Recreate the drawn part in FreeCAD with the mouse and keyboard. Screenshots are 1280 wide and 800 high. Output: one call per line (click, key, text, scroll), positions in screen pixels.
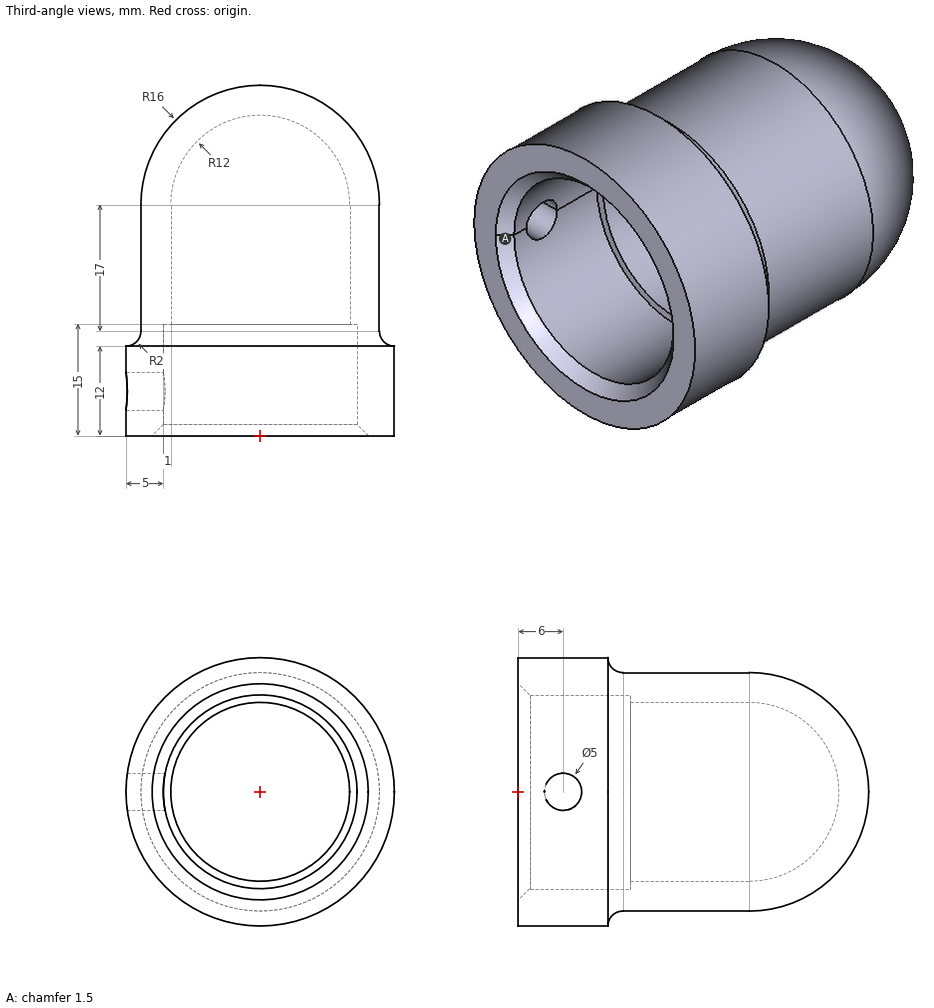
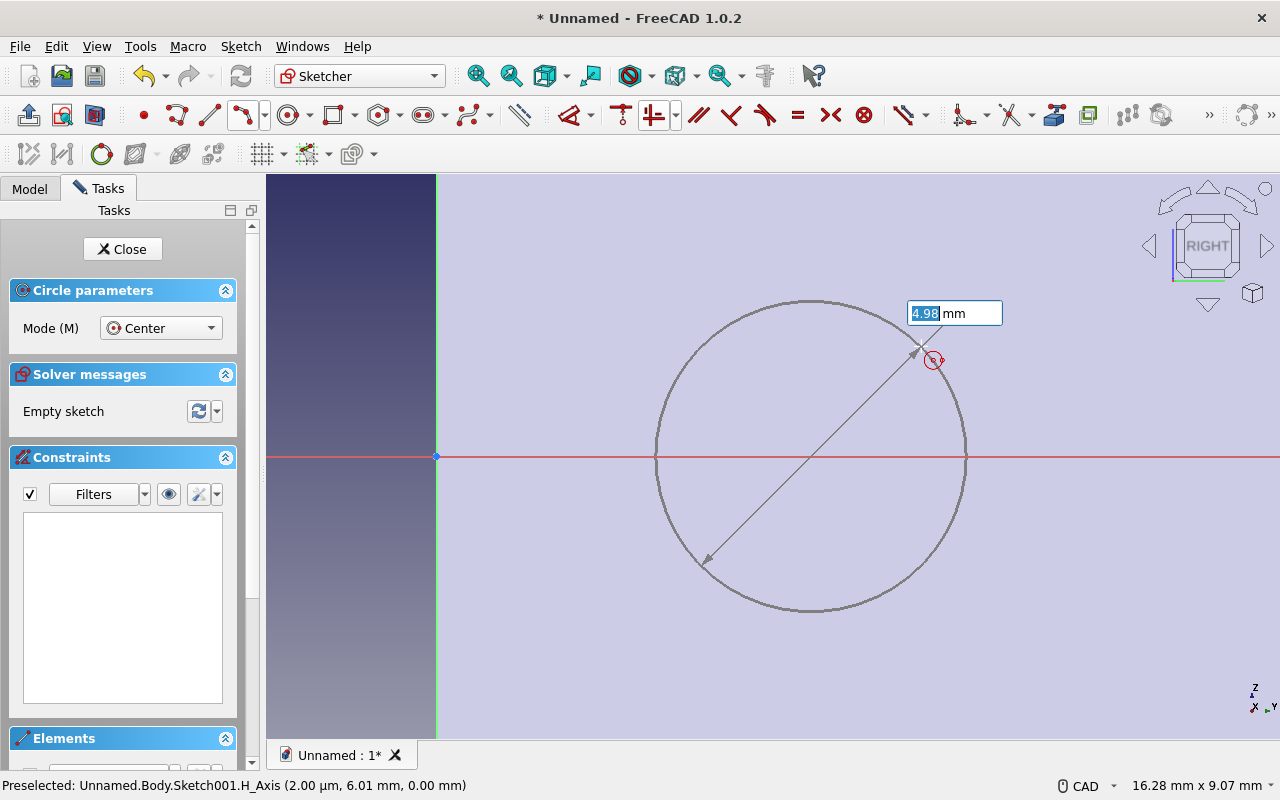
text(5)
key(Return)
key(Escape)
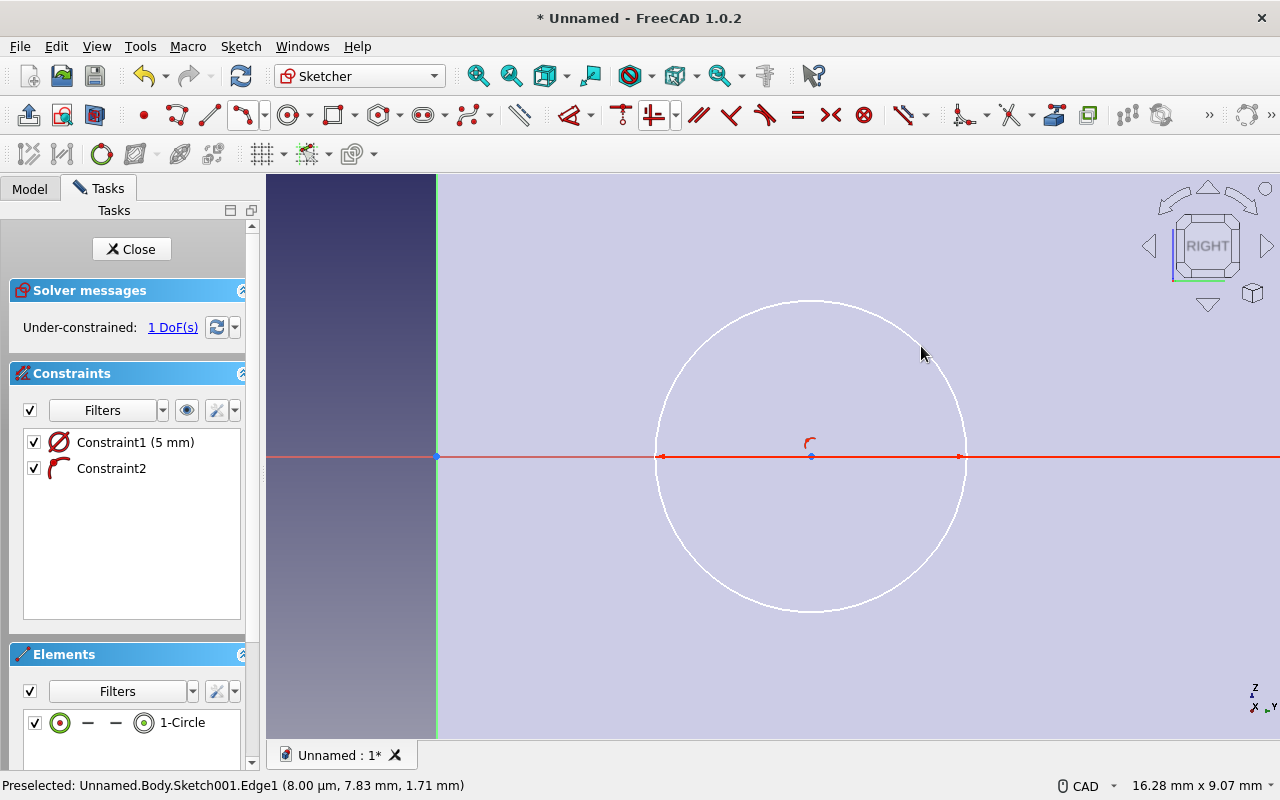
click(568, 116)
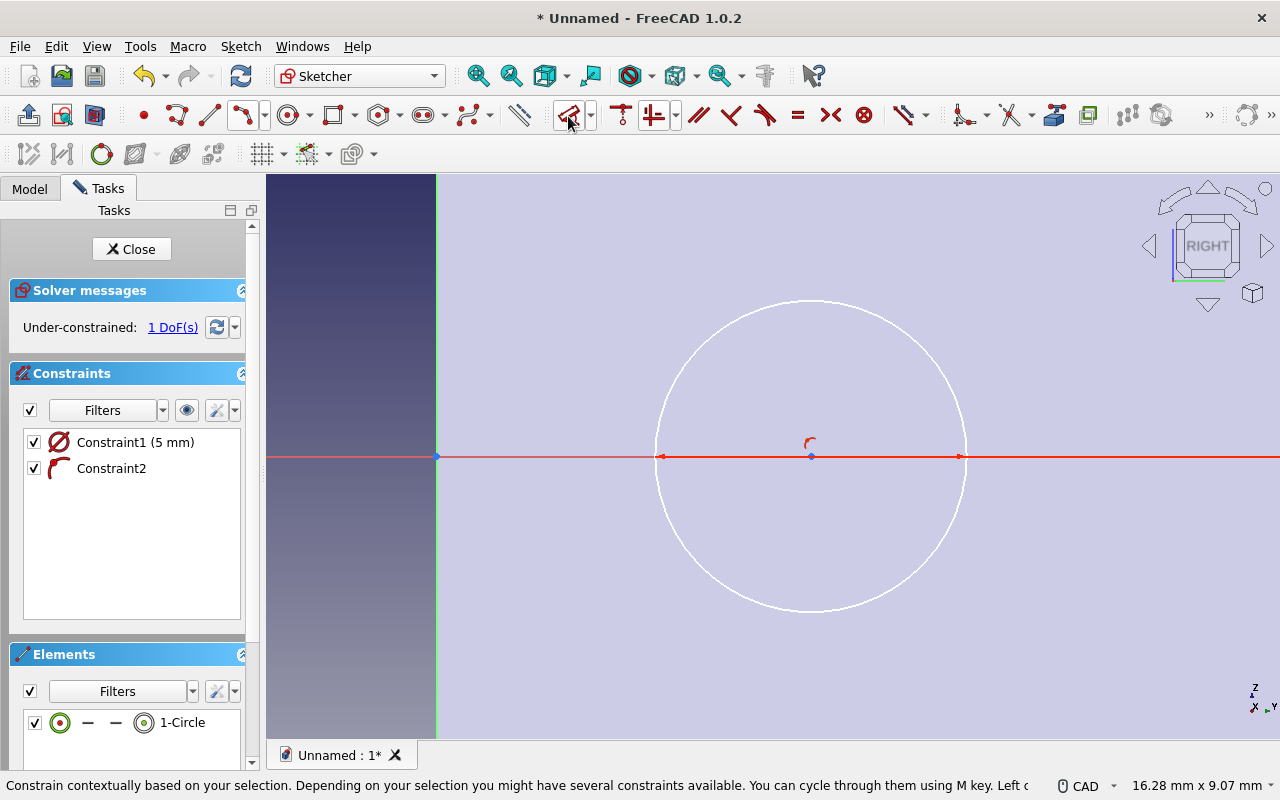
click(811, 456)
click(624, 490)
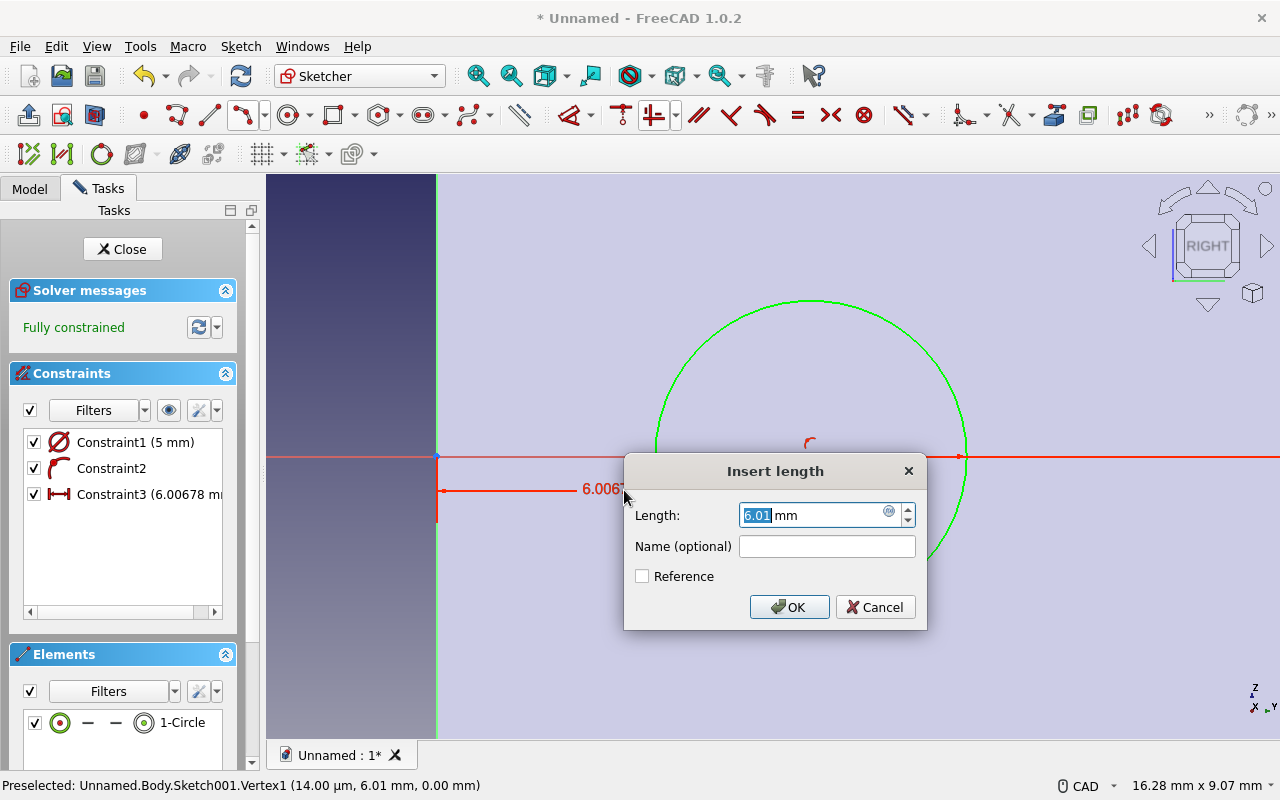
text(6)
key(Return)
key(Escape)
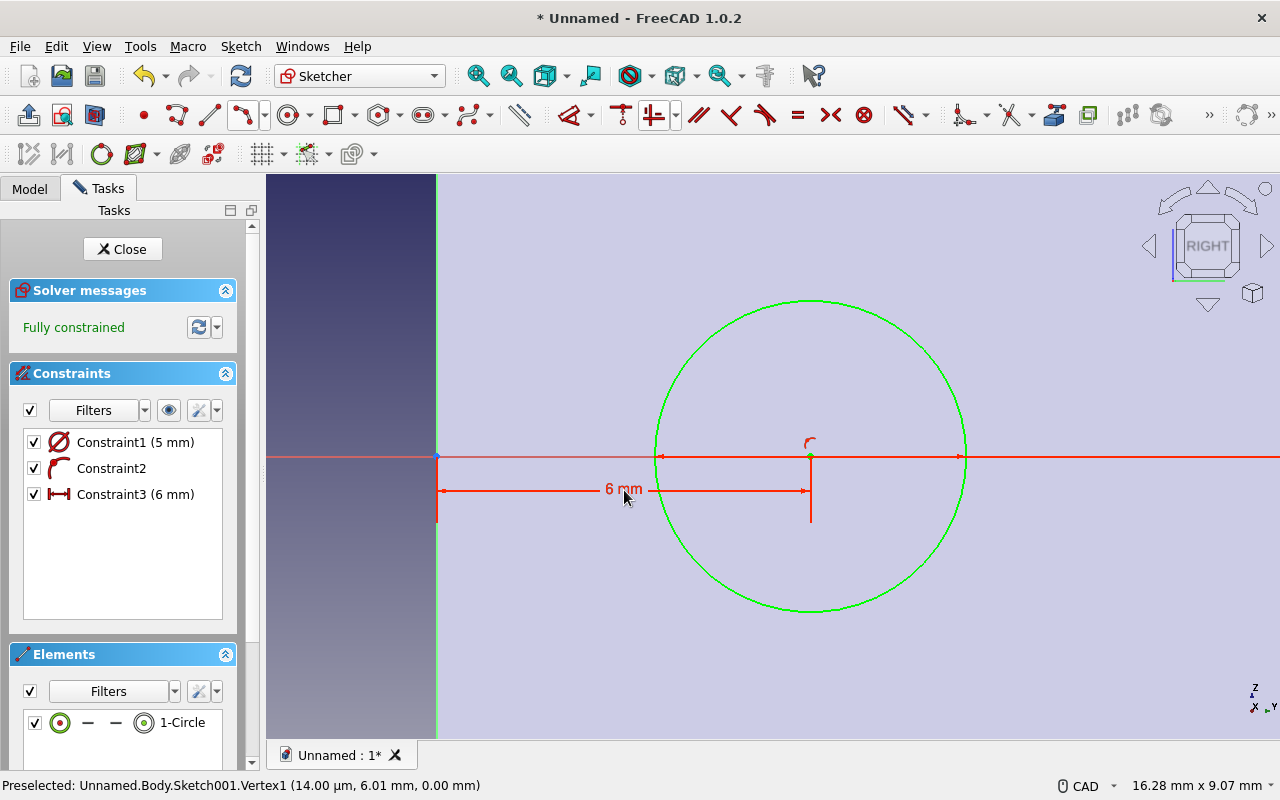
click(123, 249)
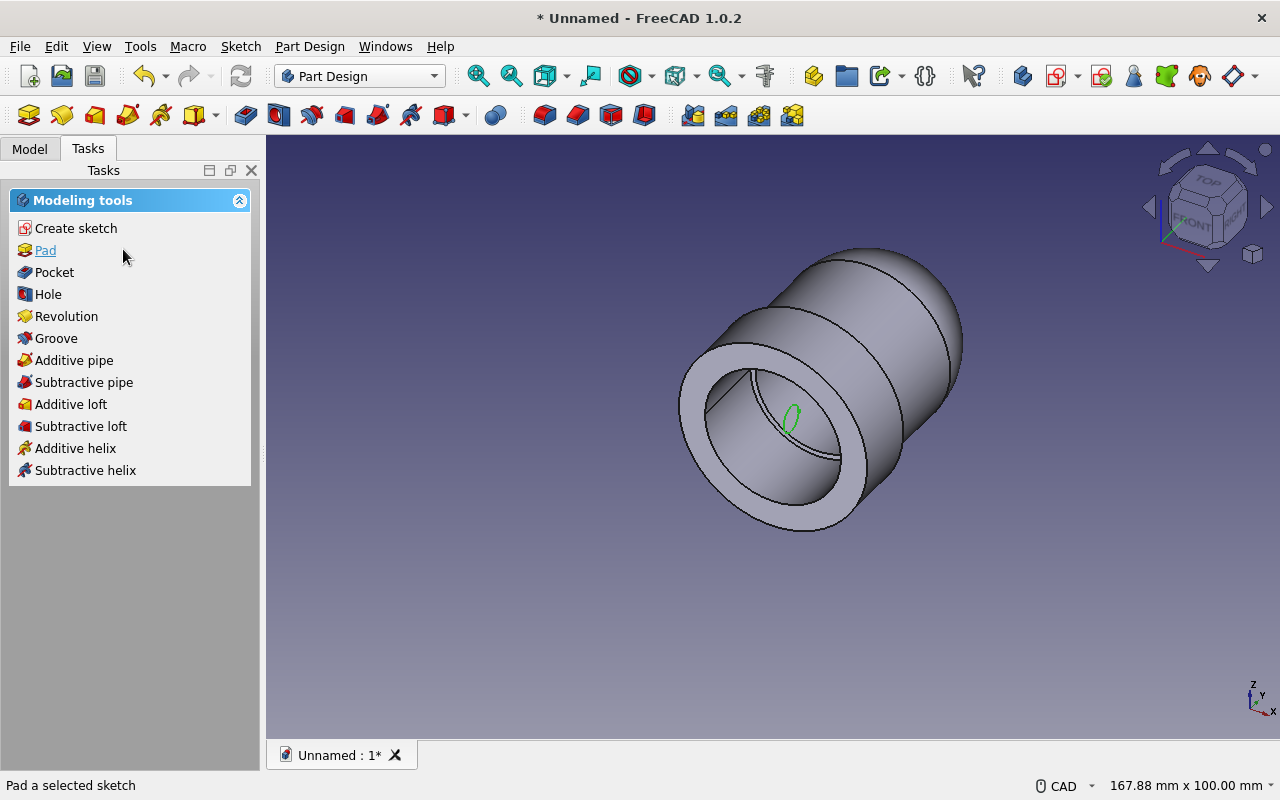
click(246, 116)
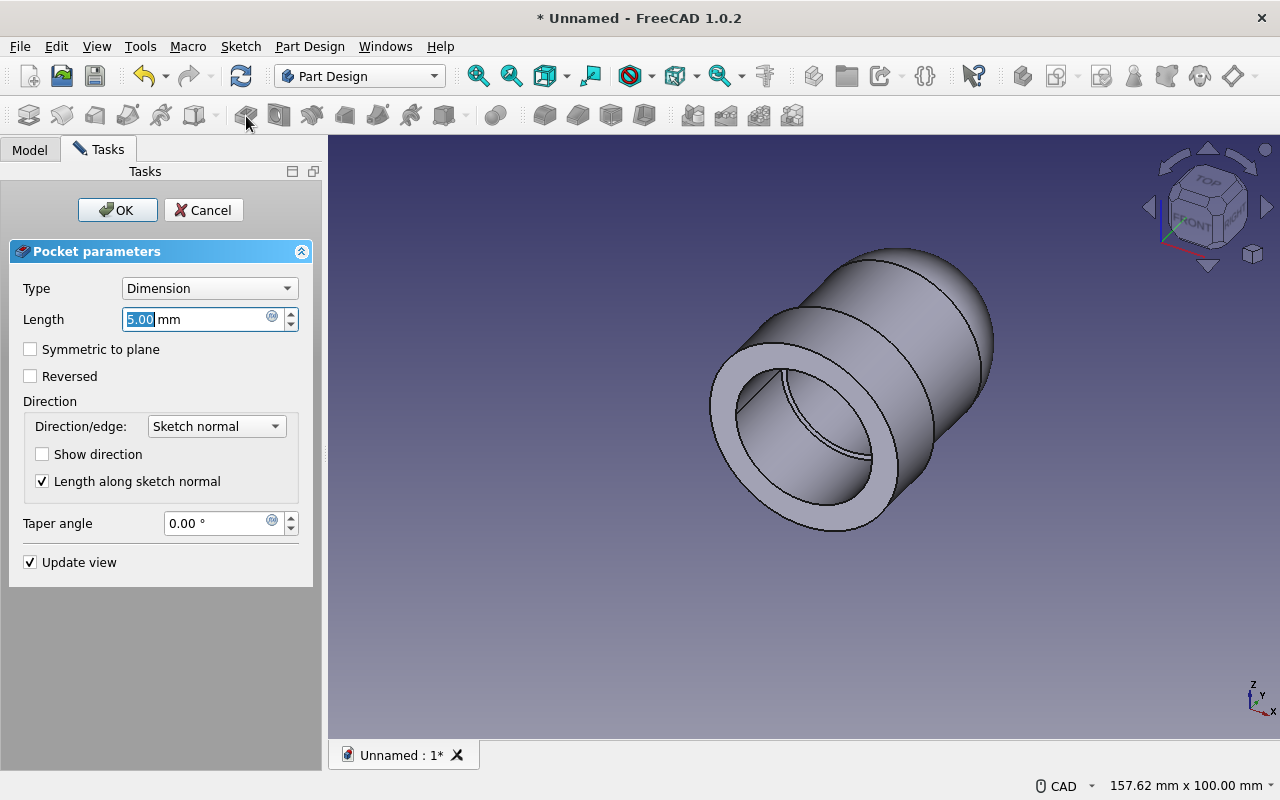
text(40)
key(Tab)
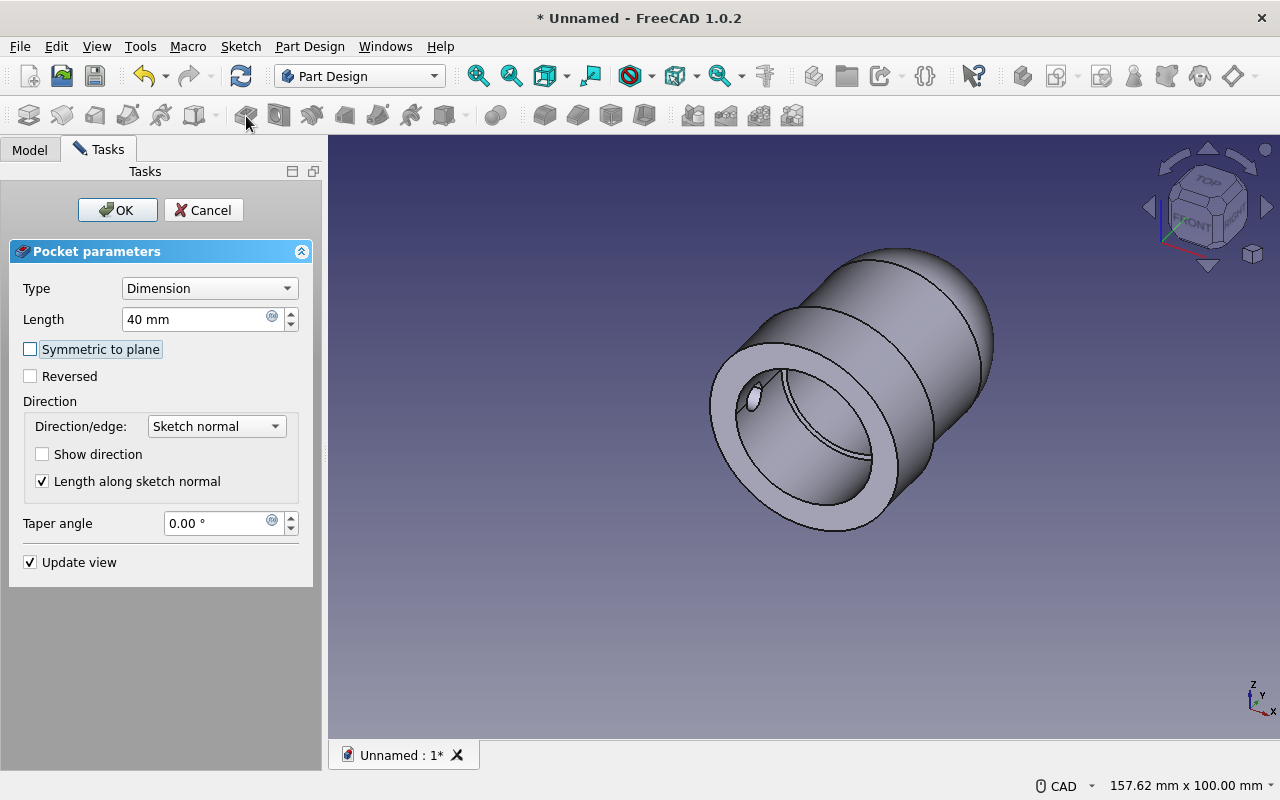
click(118, 210)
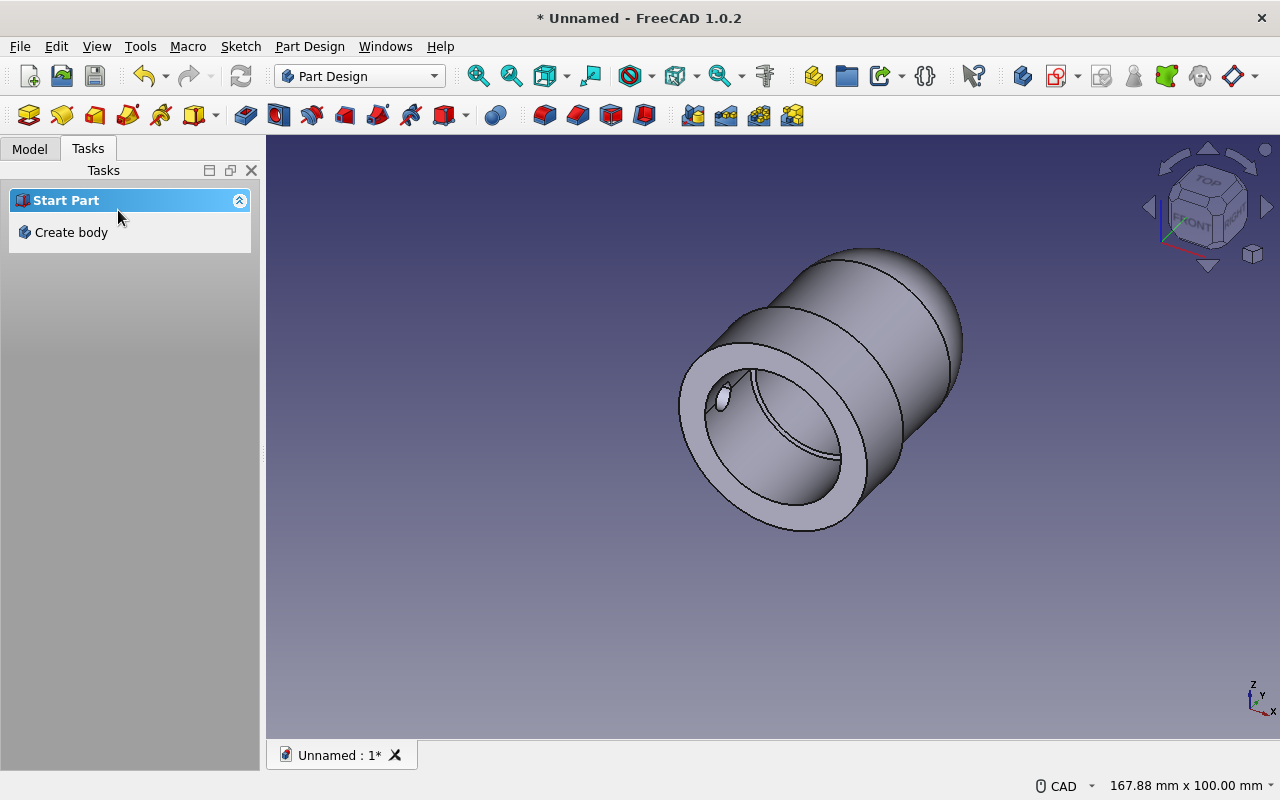
click(794, 504)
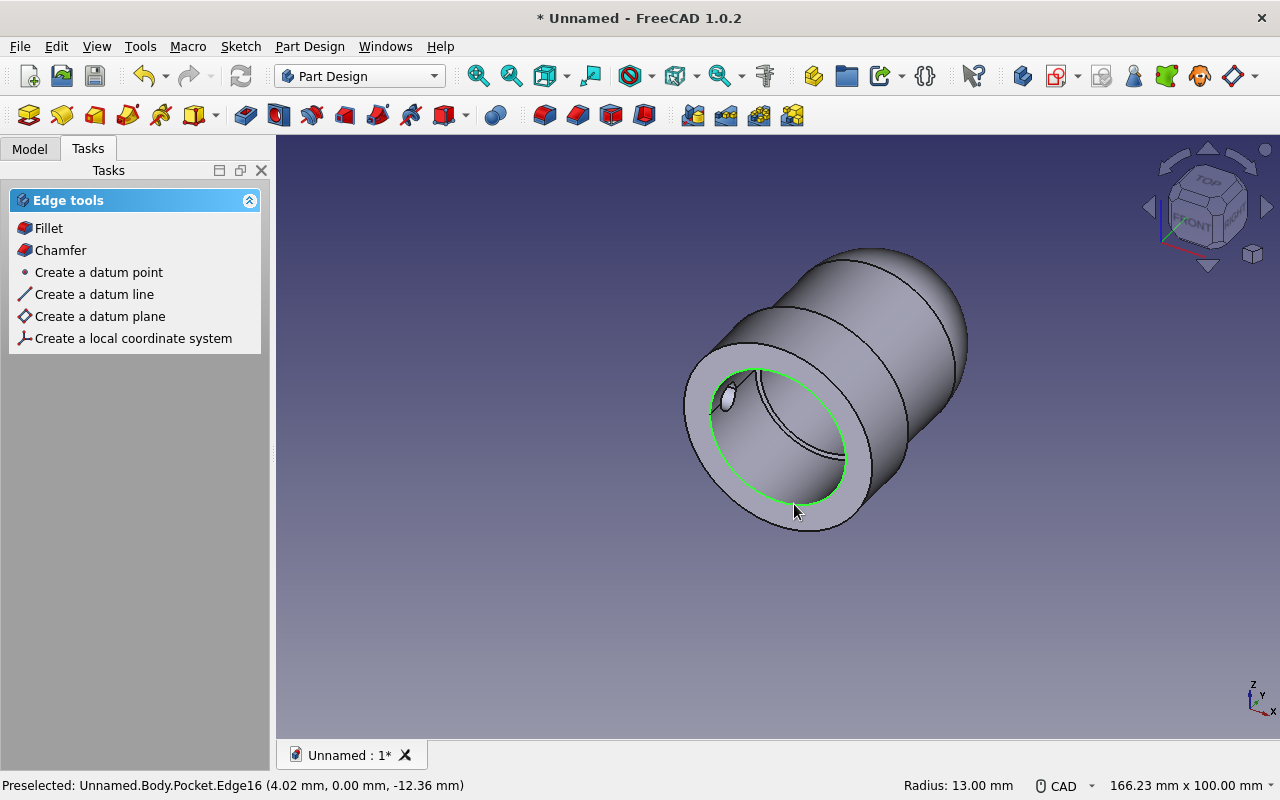
click(578, 116)